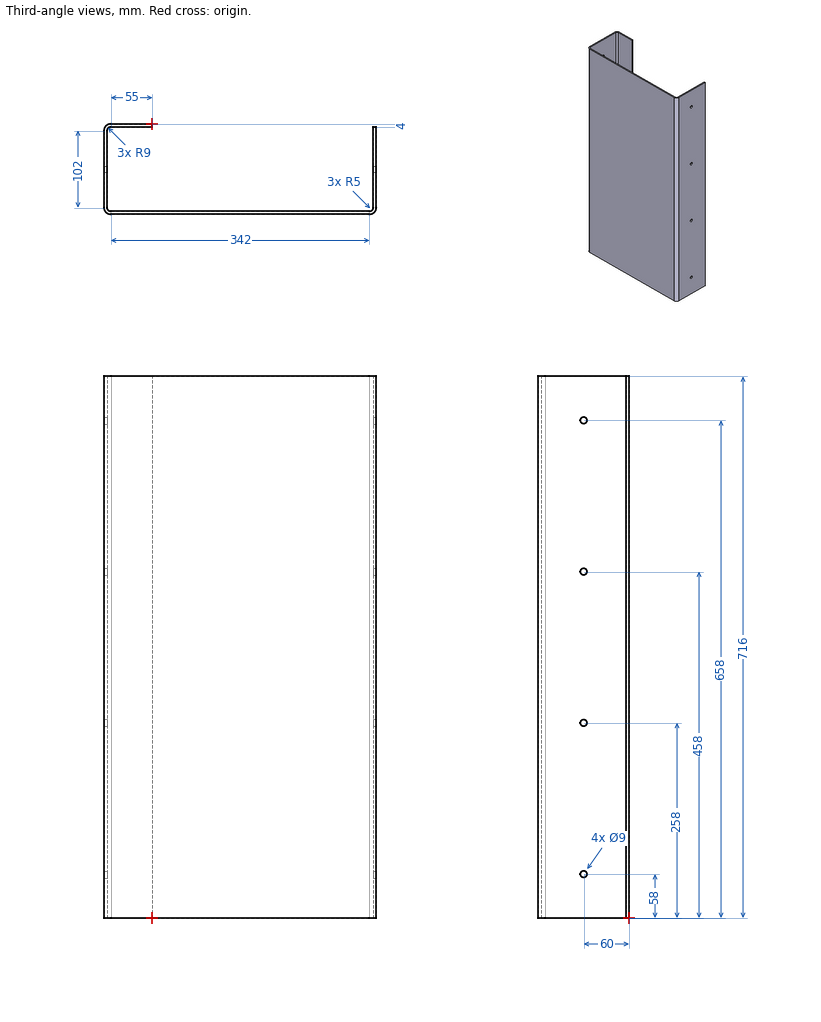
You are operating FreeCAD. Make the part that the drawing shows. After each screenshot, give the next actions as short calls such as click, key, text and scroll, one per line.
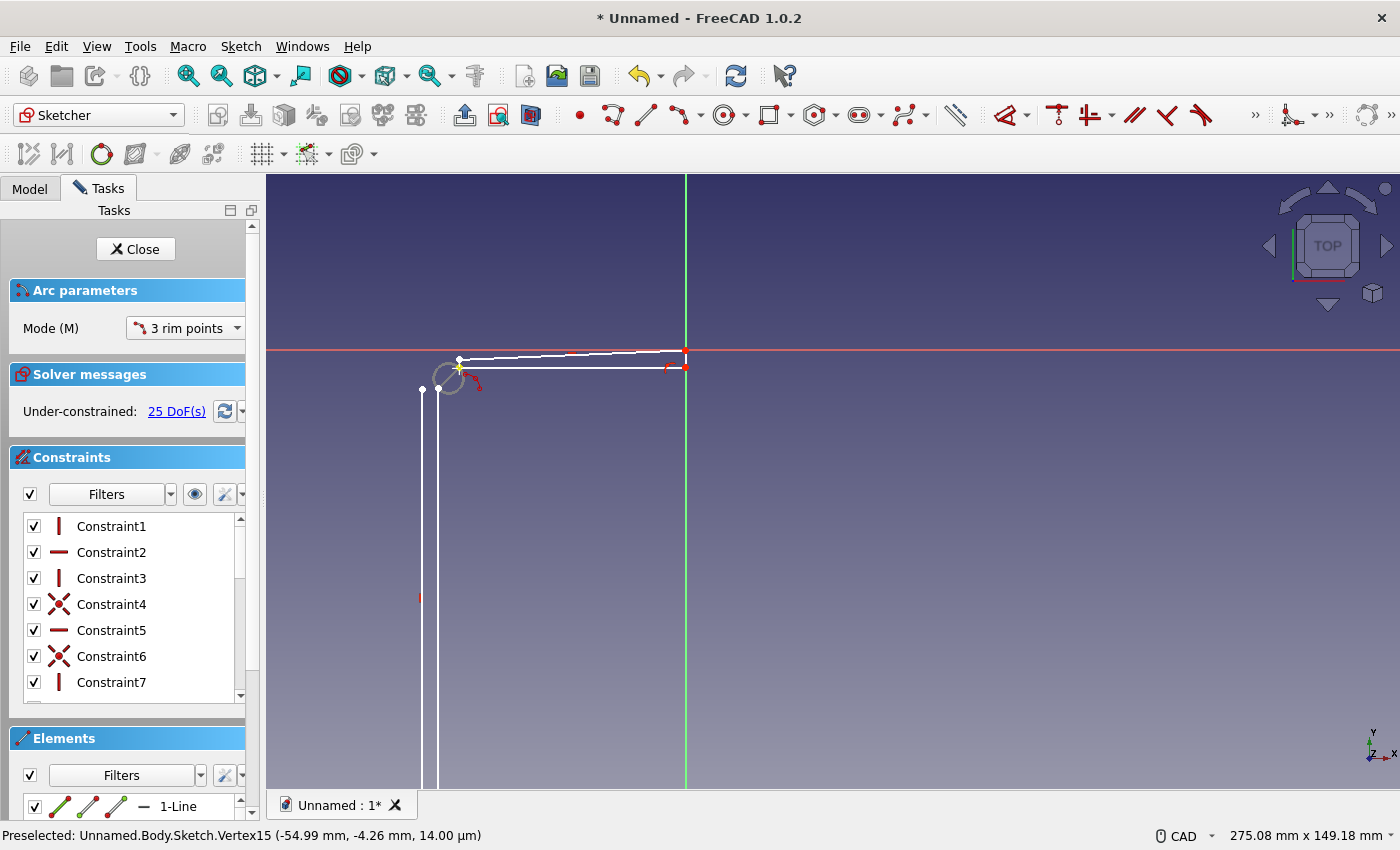
scroll(445, 373, up, 5)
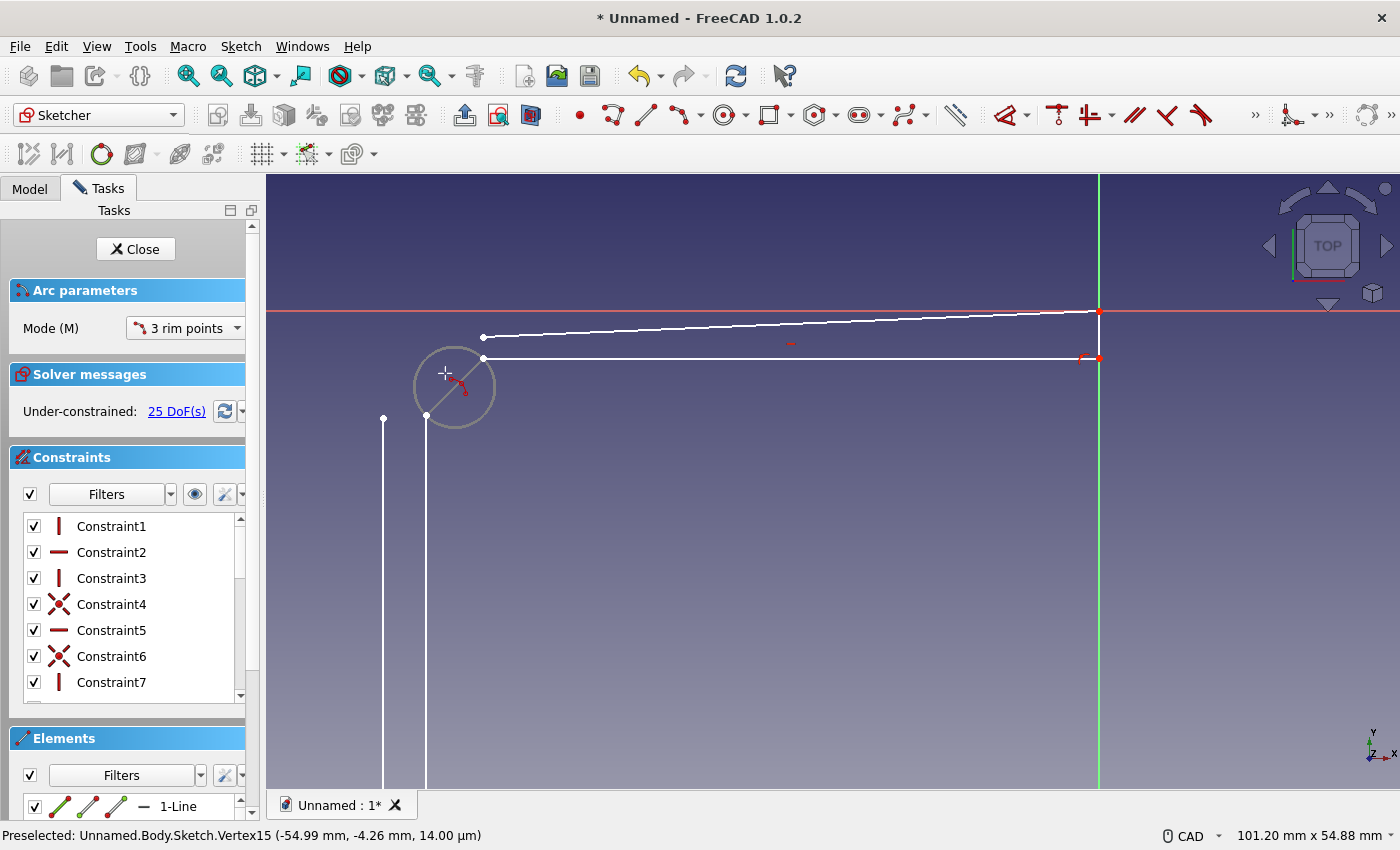
click(443, 372)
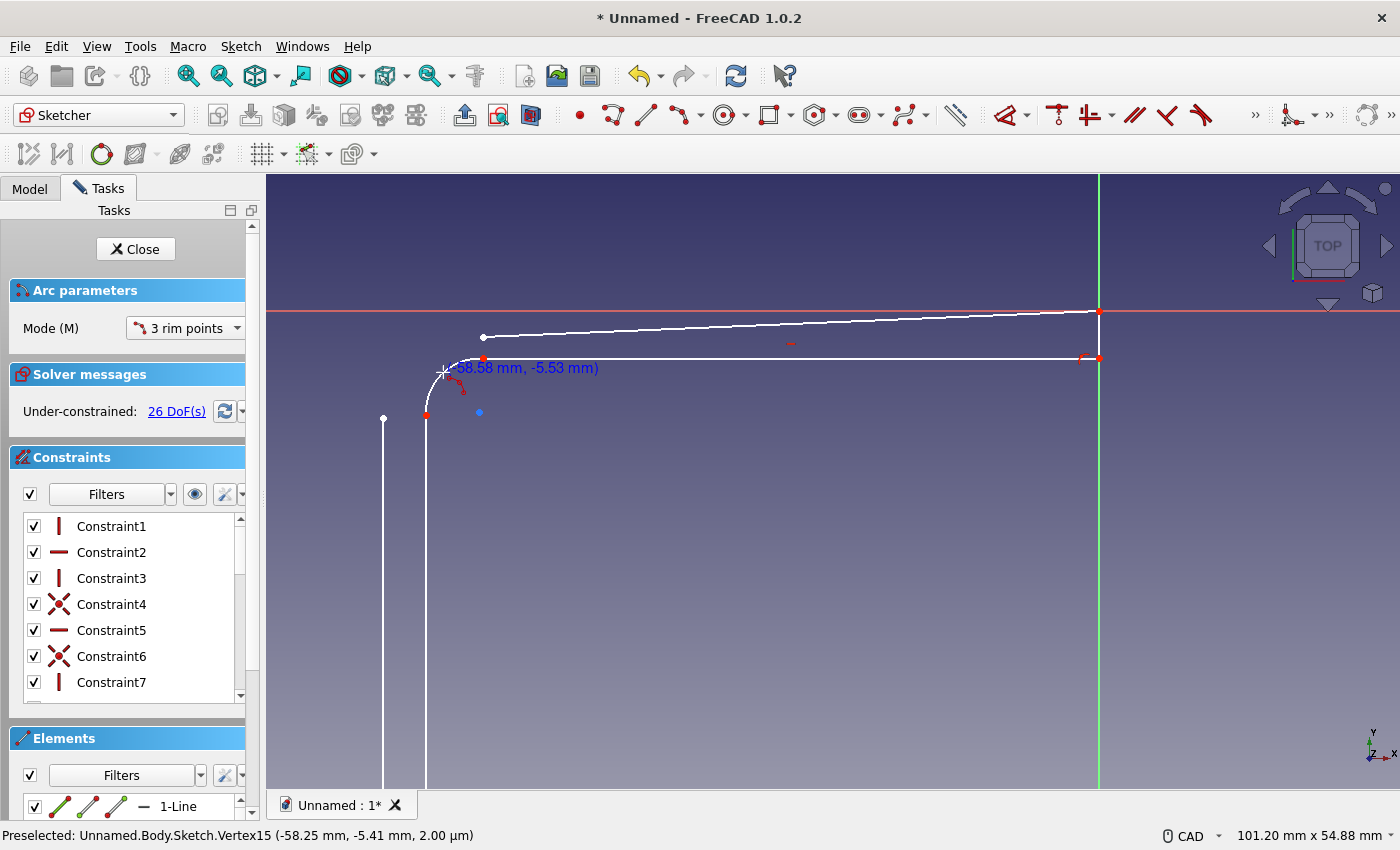
click(483, 337)
click(383, 419)
click(412, 341)
key(Escape)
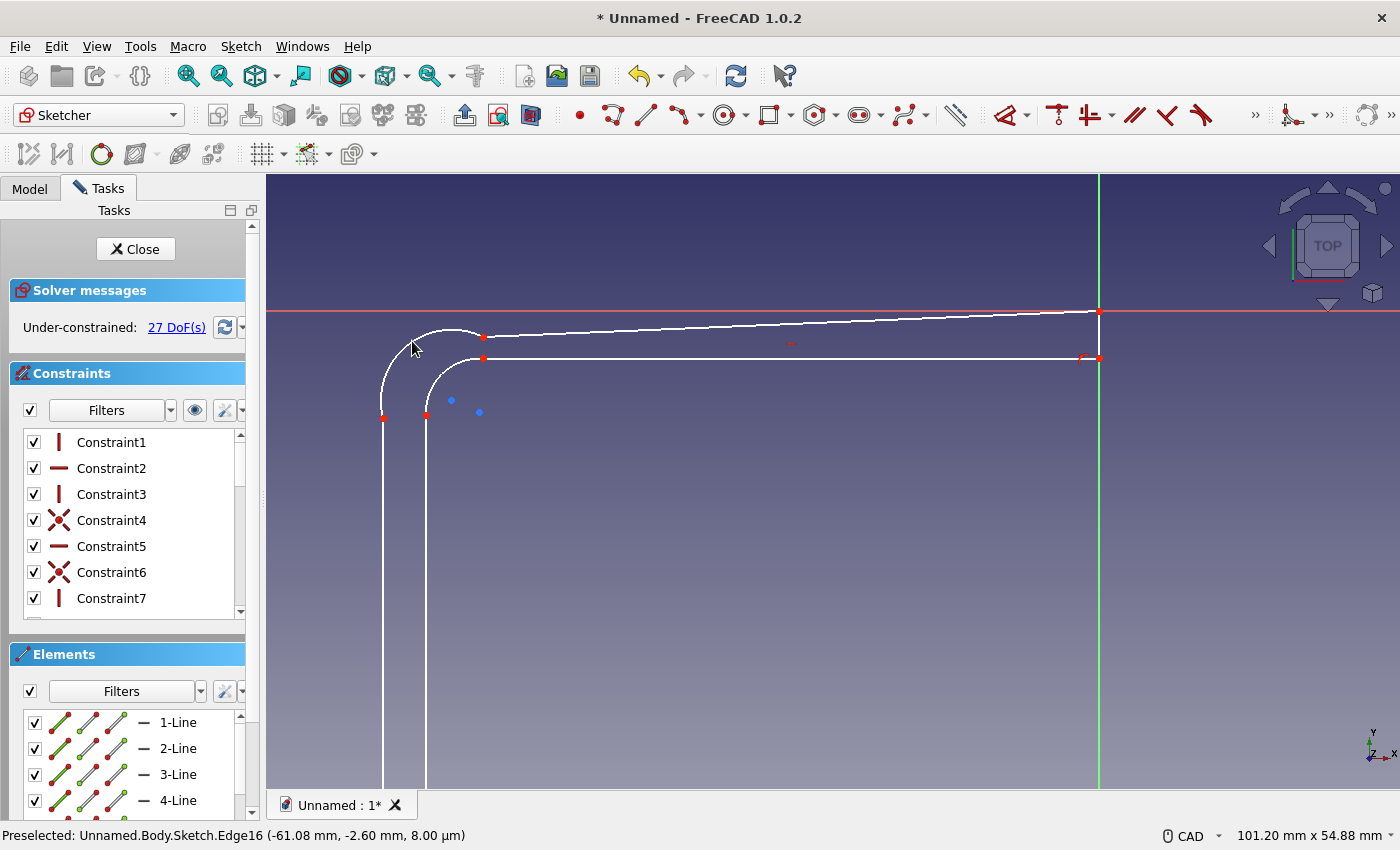
scroll(441, 382, down, 9)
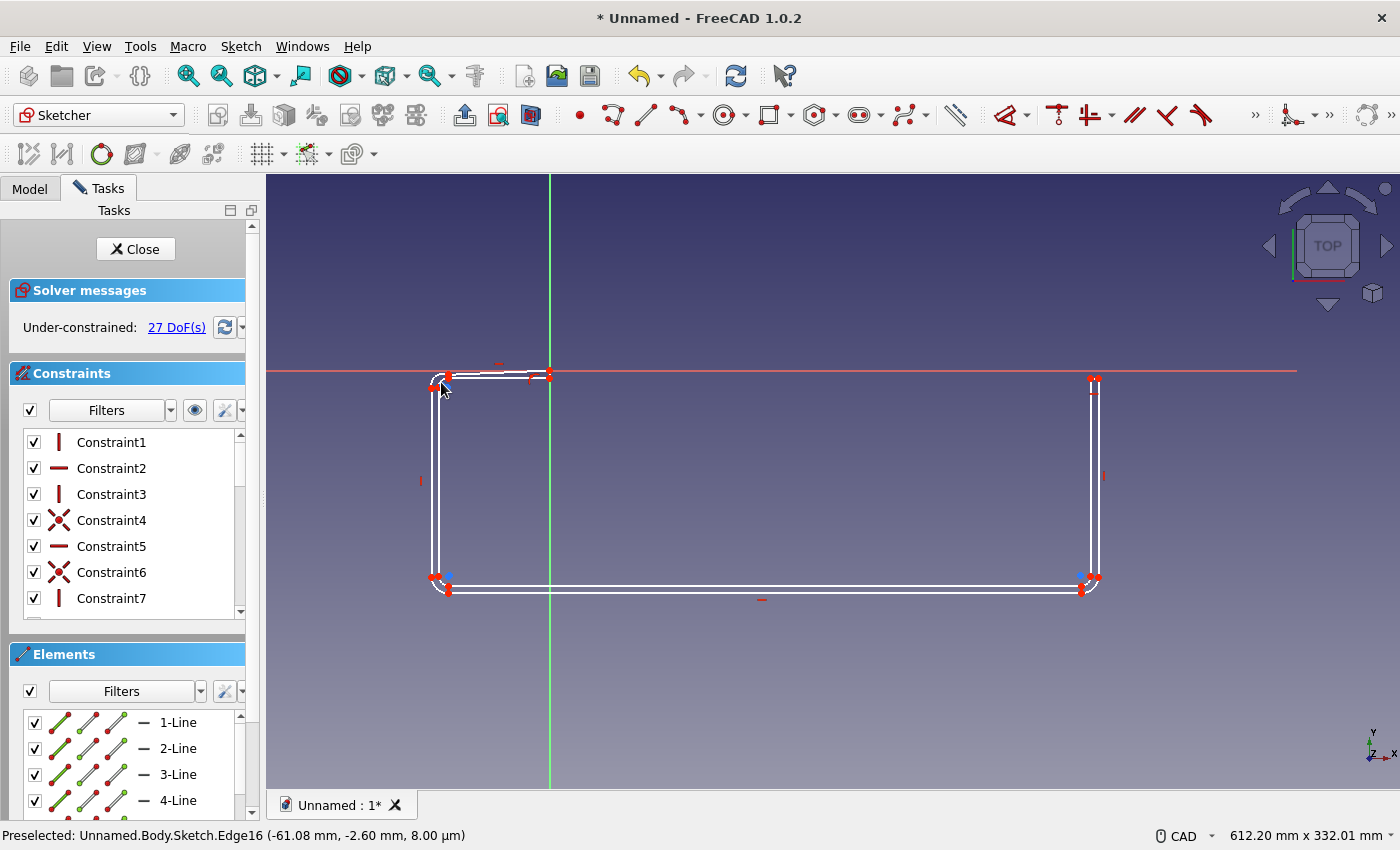
scroll(432, 426, up, 4)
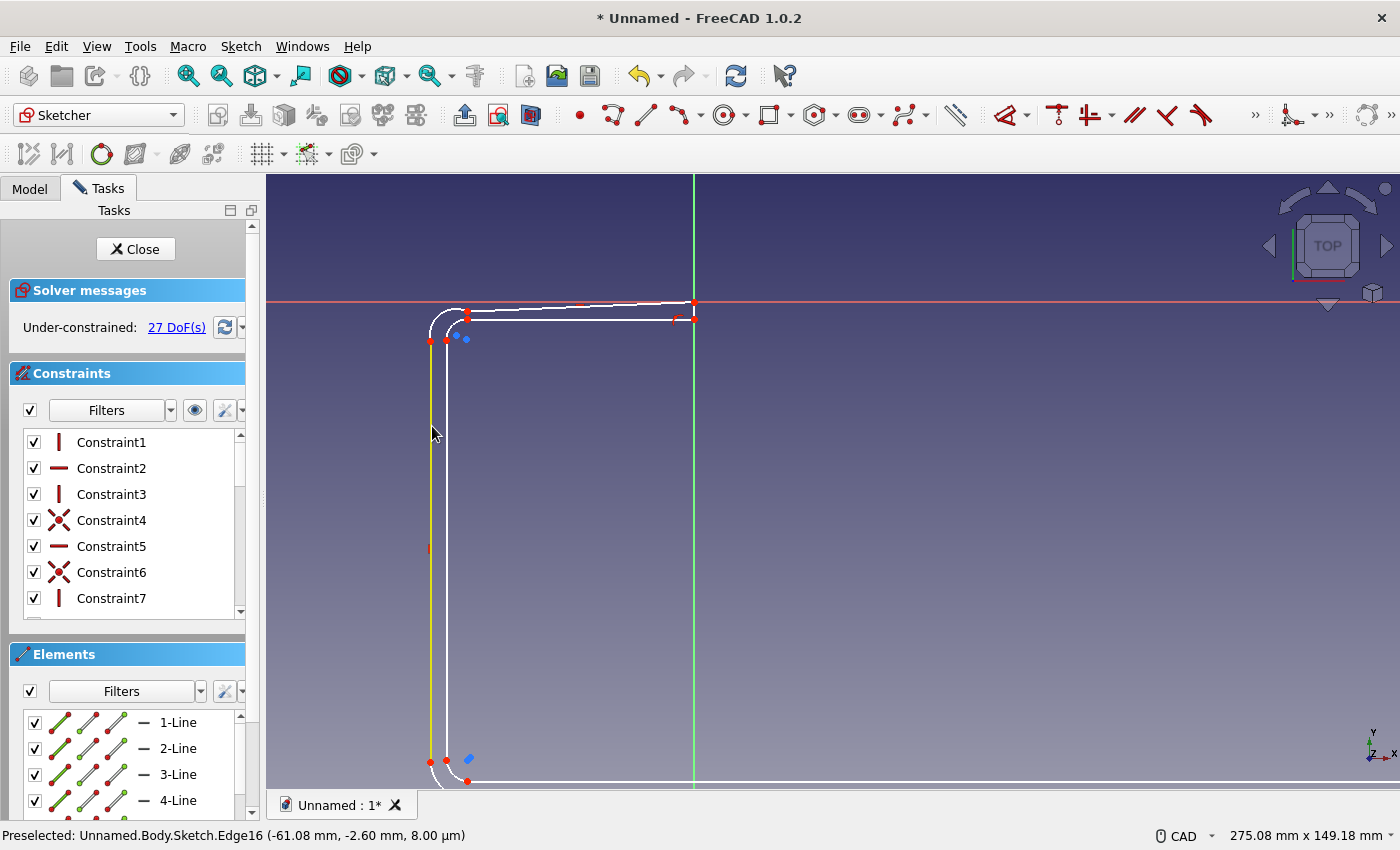
click(431, 426)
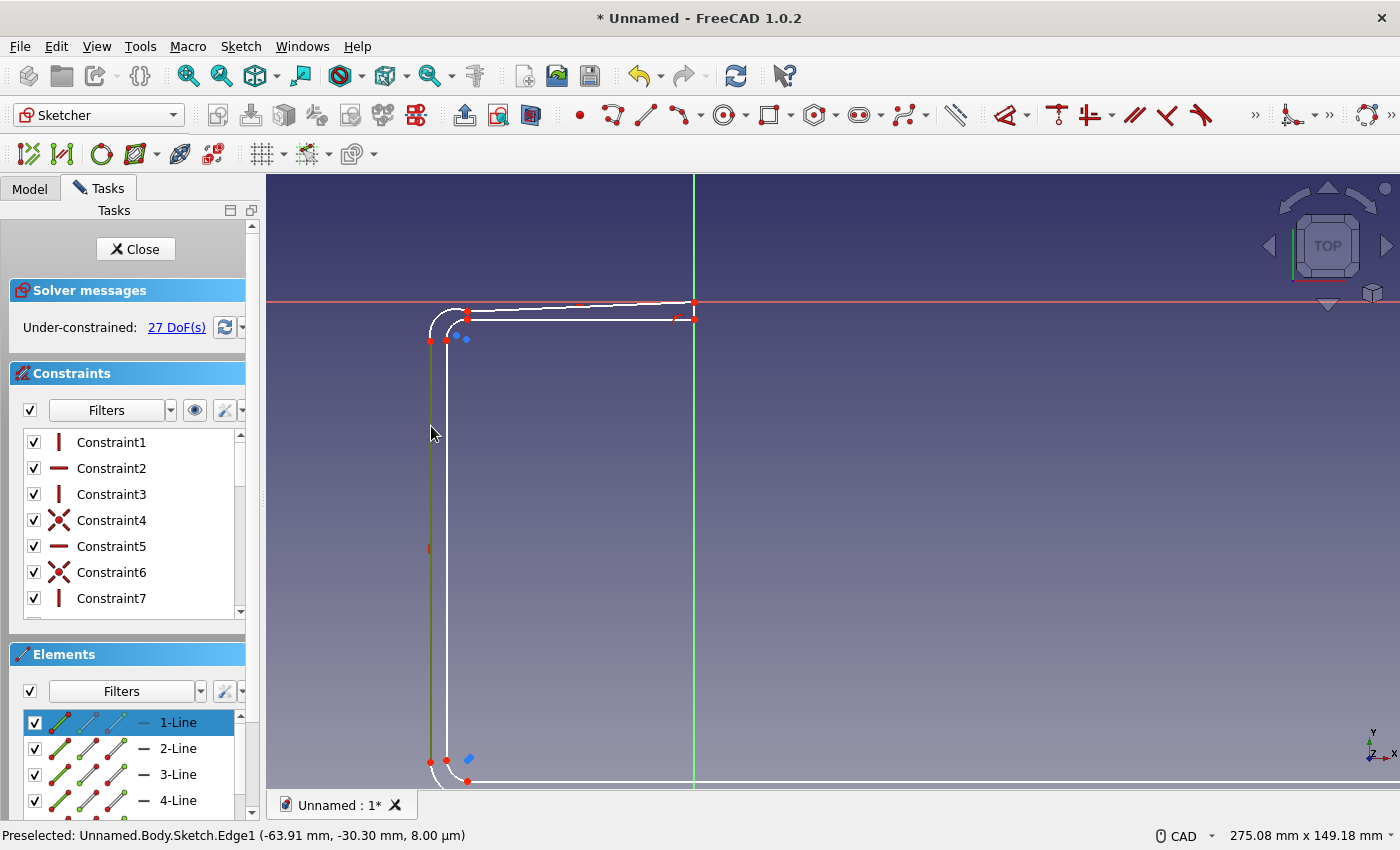
scroll(432, 426, down, 4)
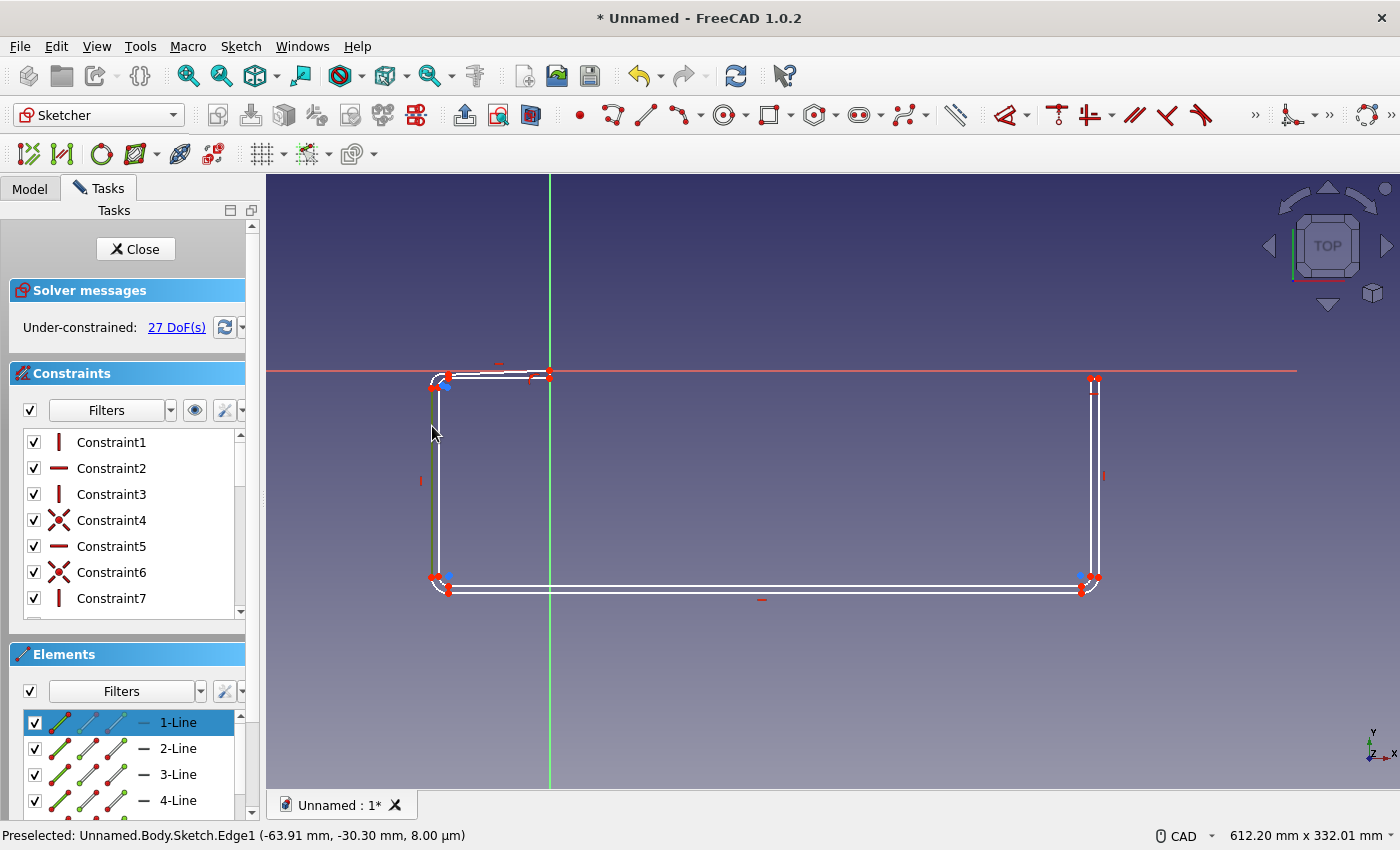
scroll(434, 585, up, 4)